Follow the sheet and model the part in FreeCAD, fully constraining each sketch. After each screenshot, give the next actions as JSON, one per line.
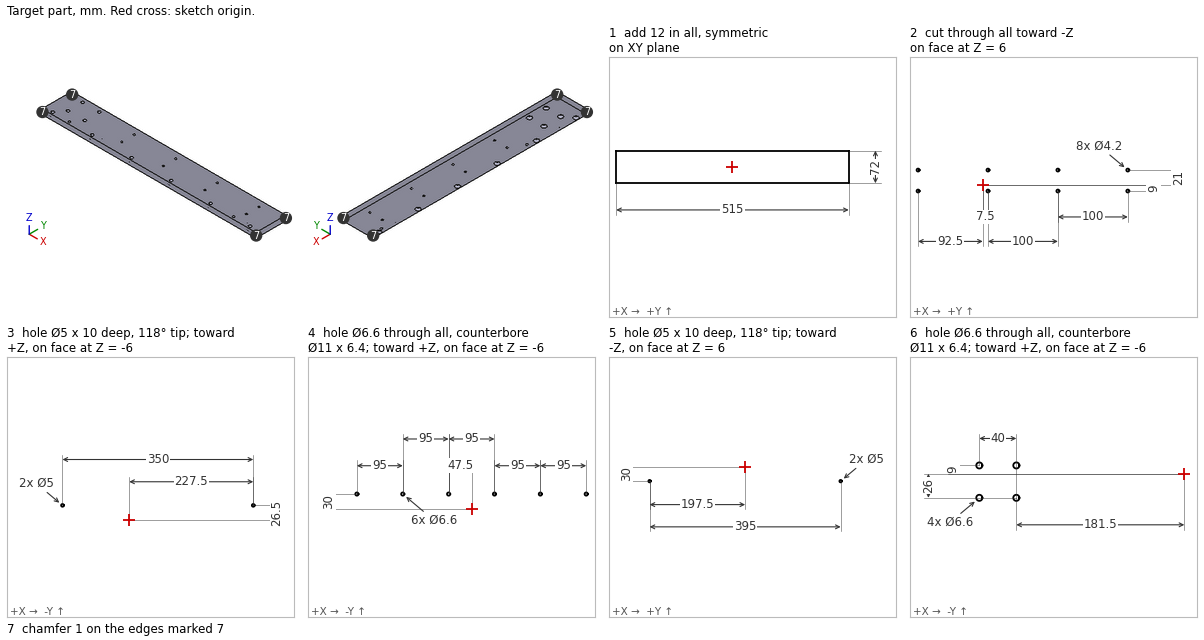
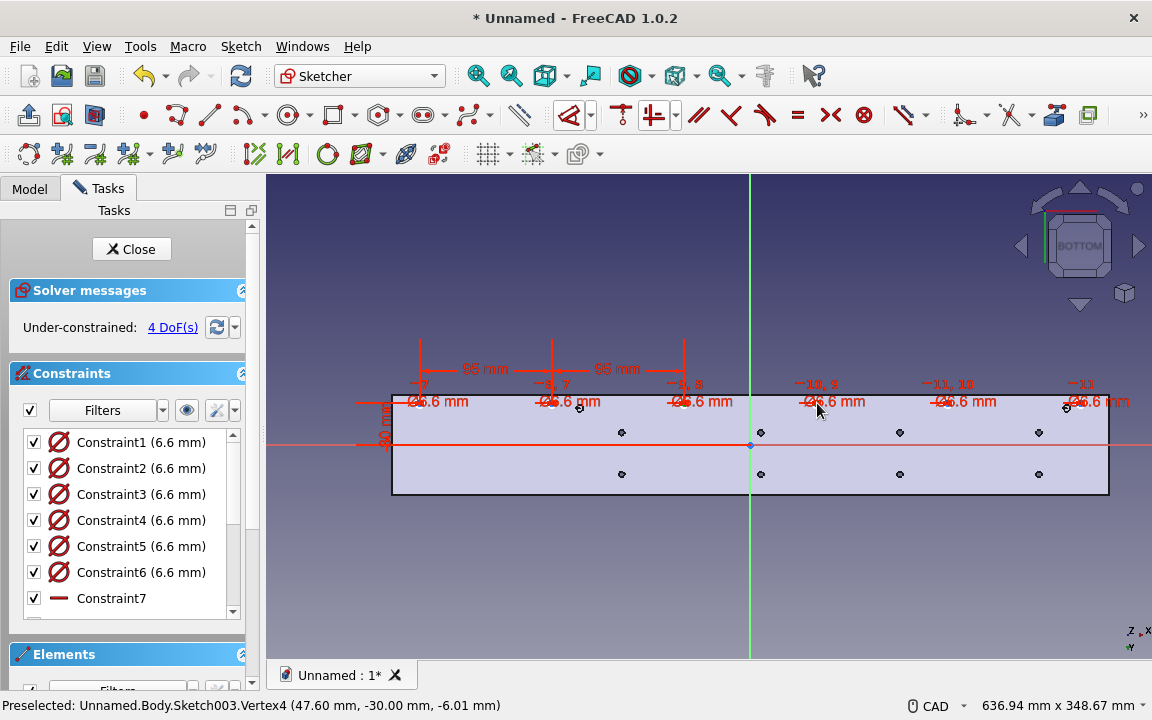
{"action": "key", "text": "l"}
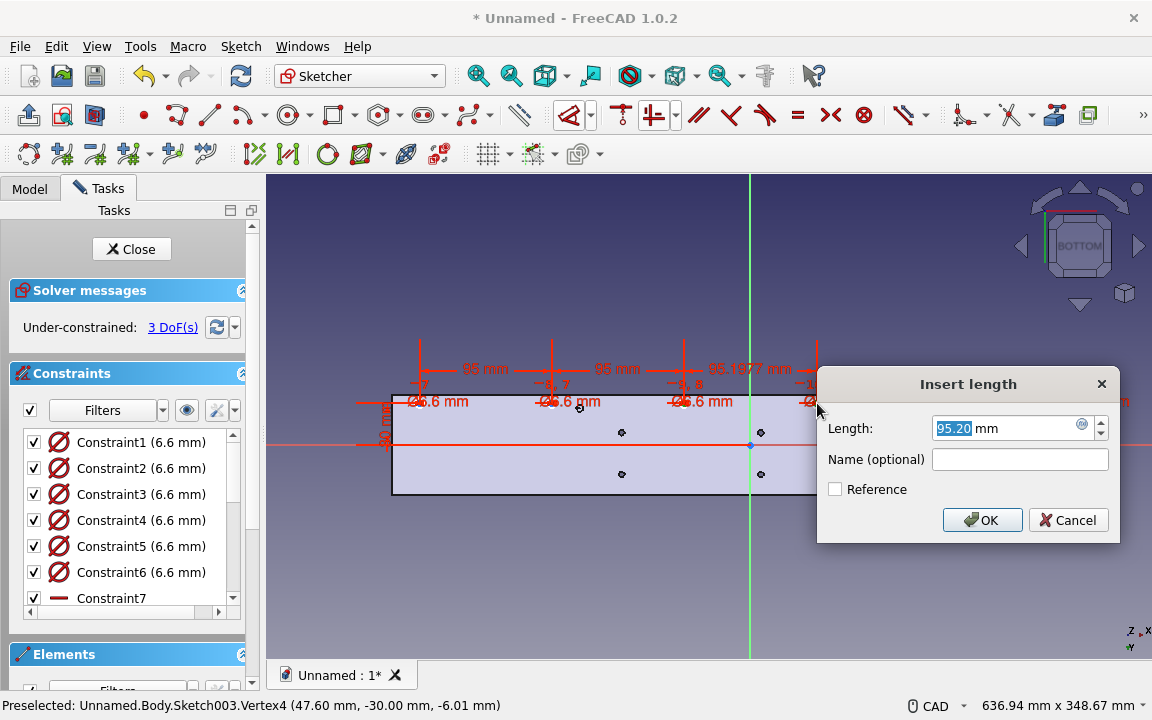
{"action": "type", "text": "95"}
{"action": "key", "text": "Return"}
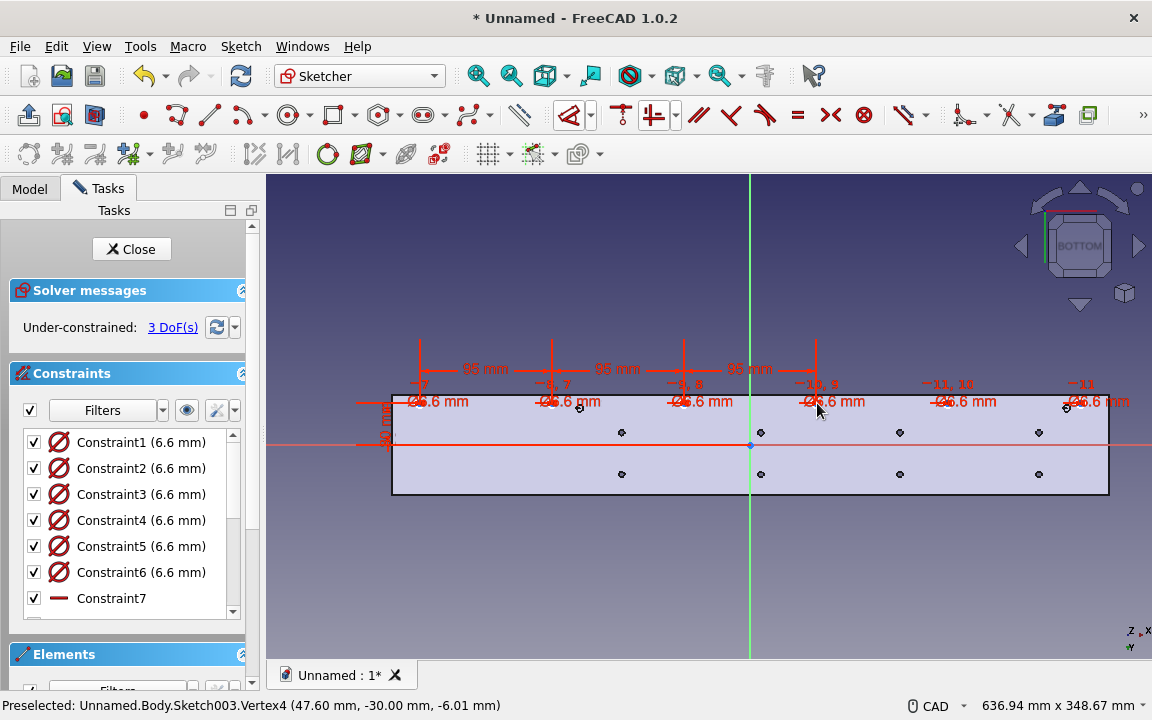
{"action": "left_click", "coordinate": [816, 403]}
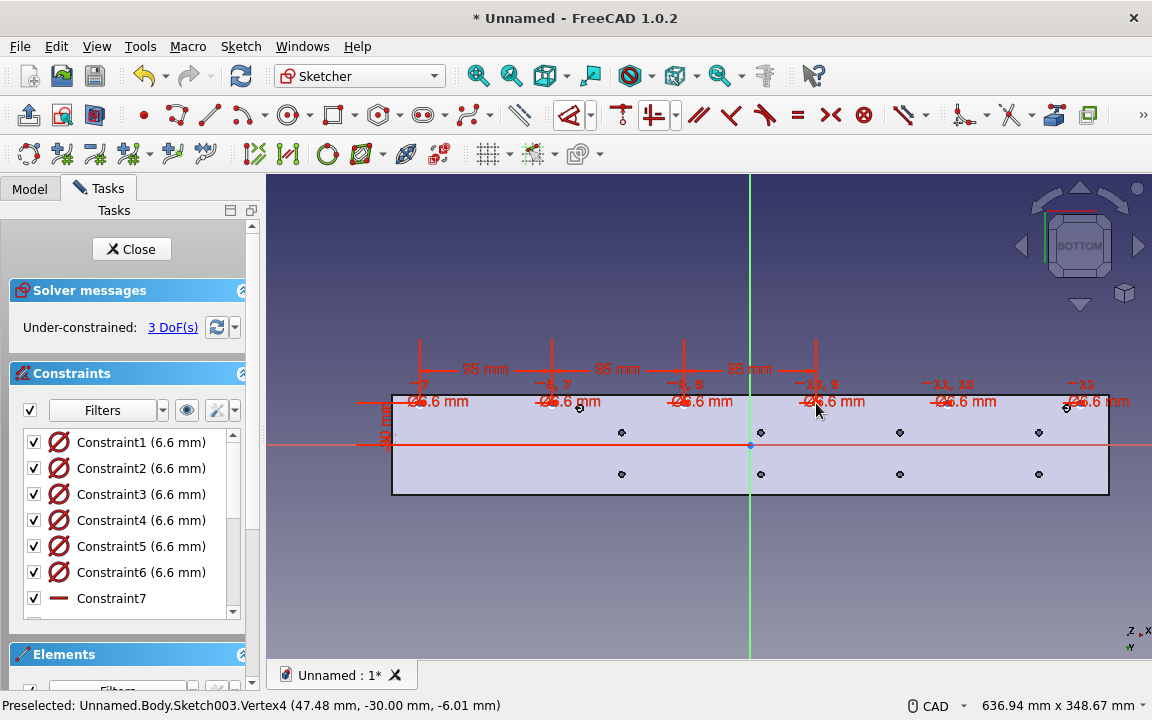
{"action": "left_click", "coordinate": [948, 403]}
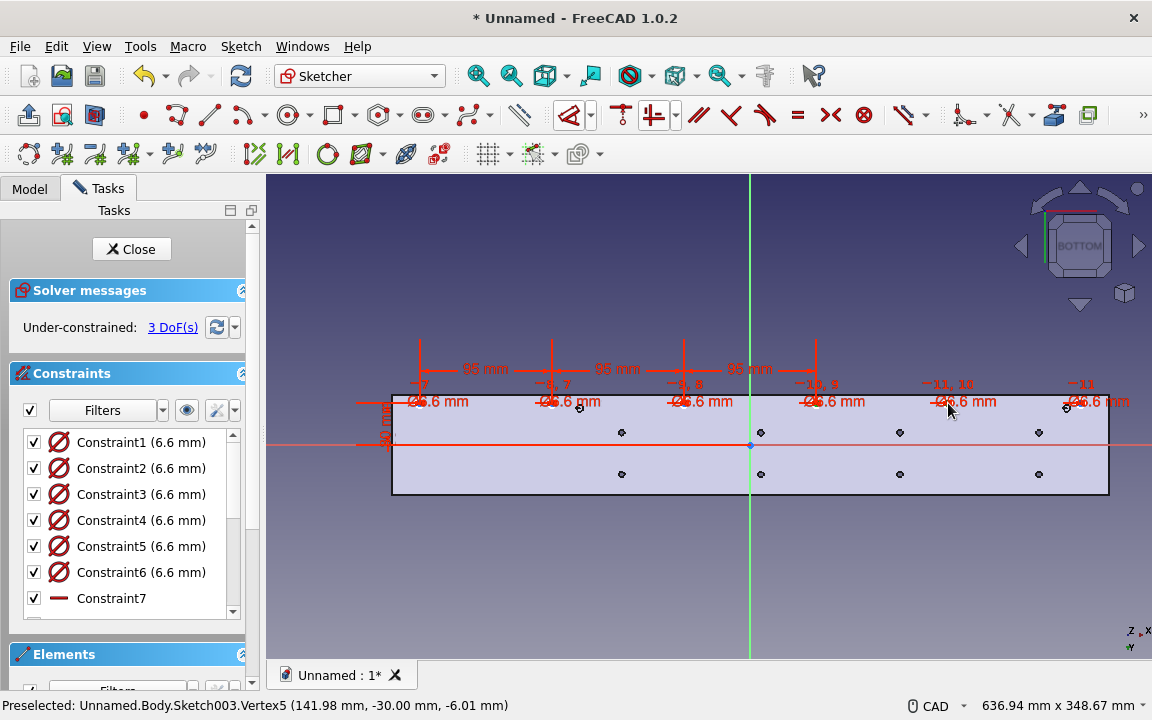
{"action": "key", "text": "l"}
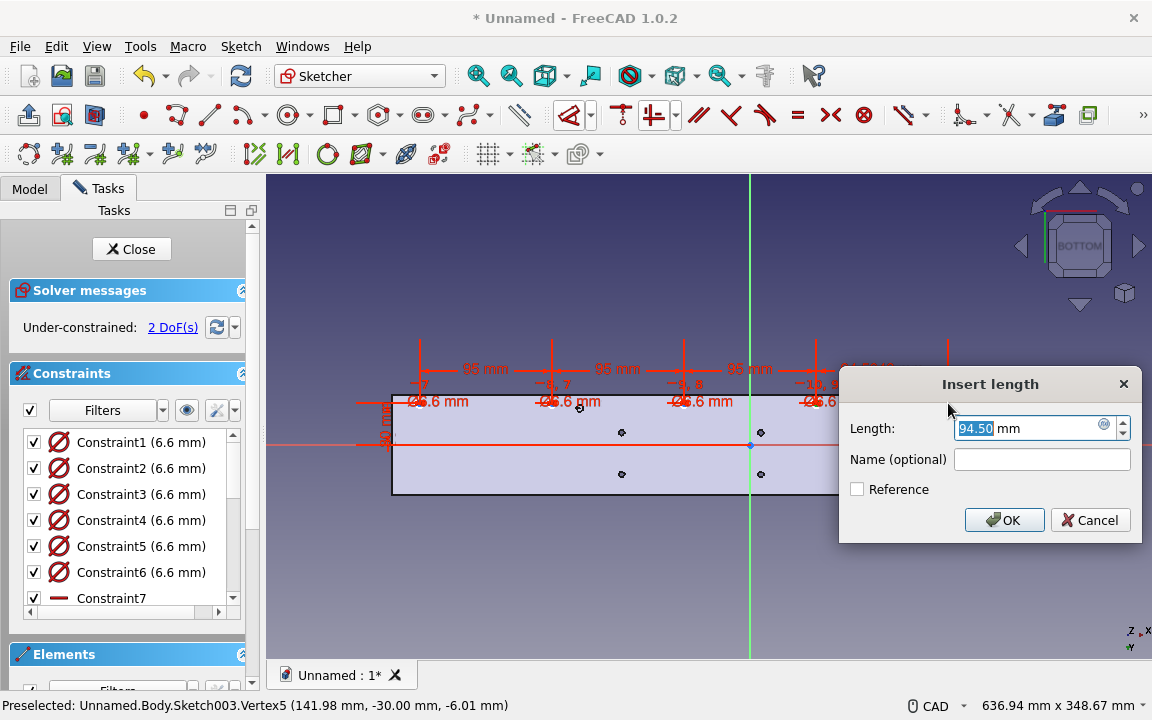
{"action": "type", "text": "95"}
{"action": "key", "text": "Return"}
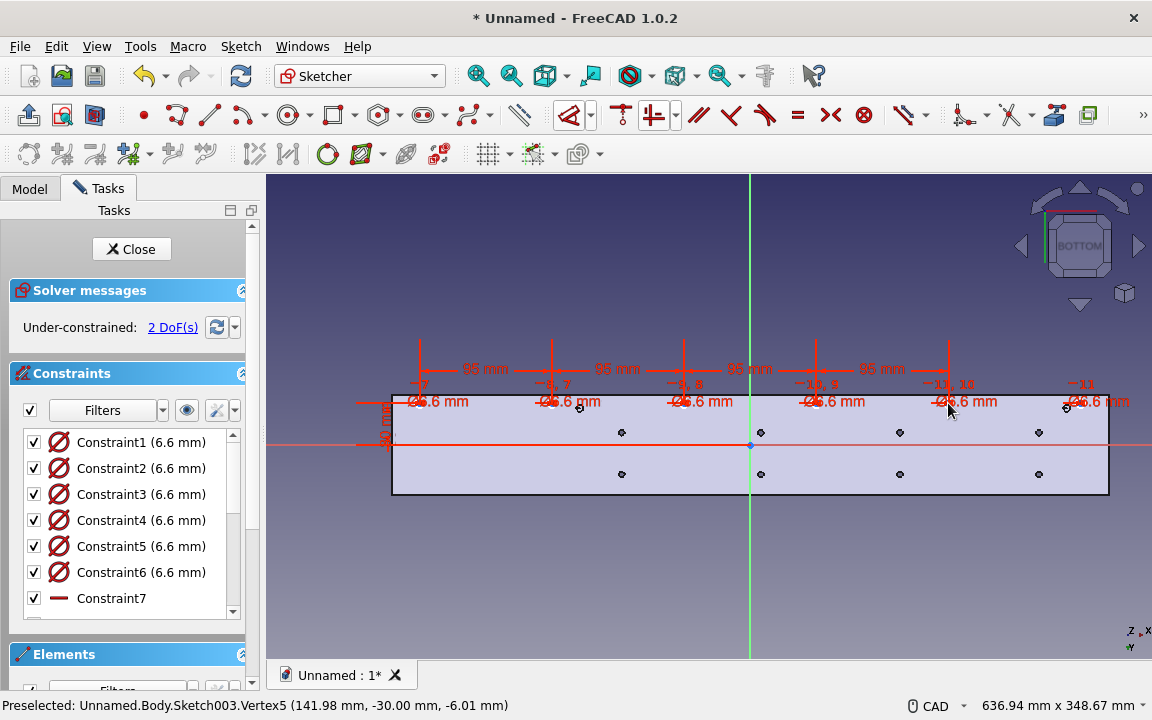
{"action": "left_click", "coordinate": [949, 403]}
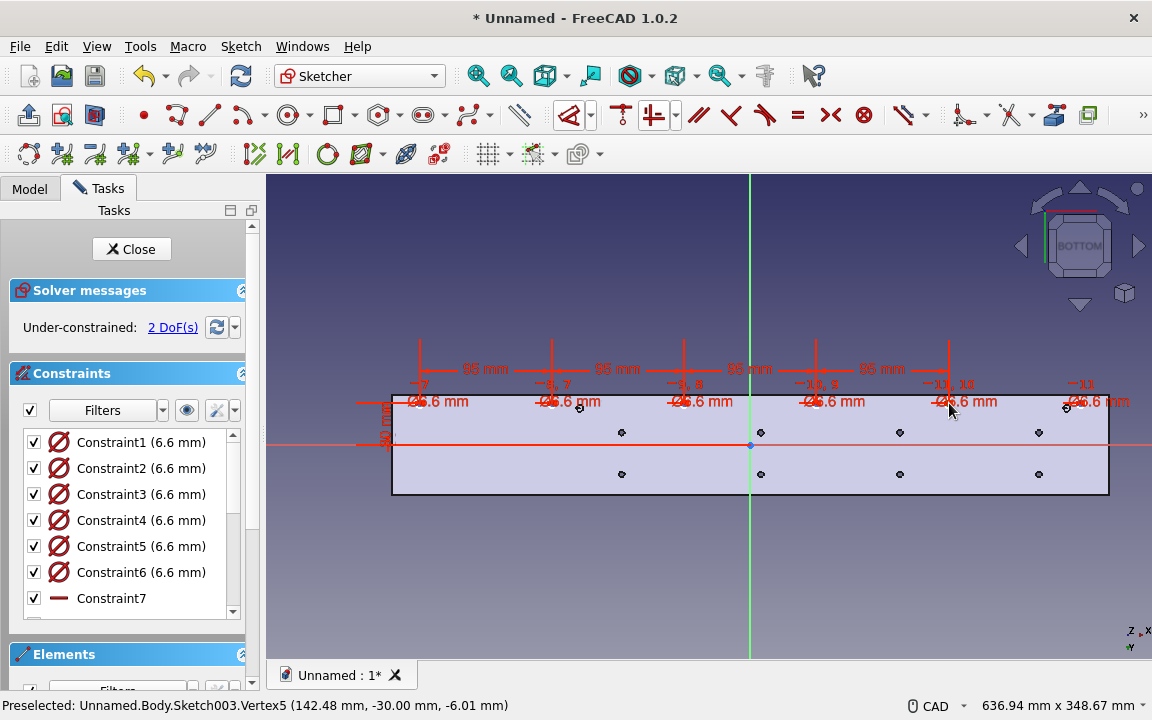
{"action": "scroll", "coordinate": [417, 405], "scroll_direction": "down", "scroll_amount": 2}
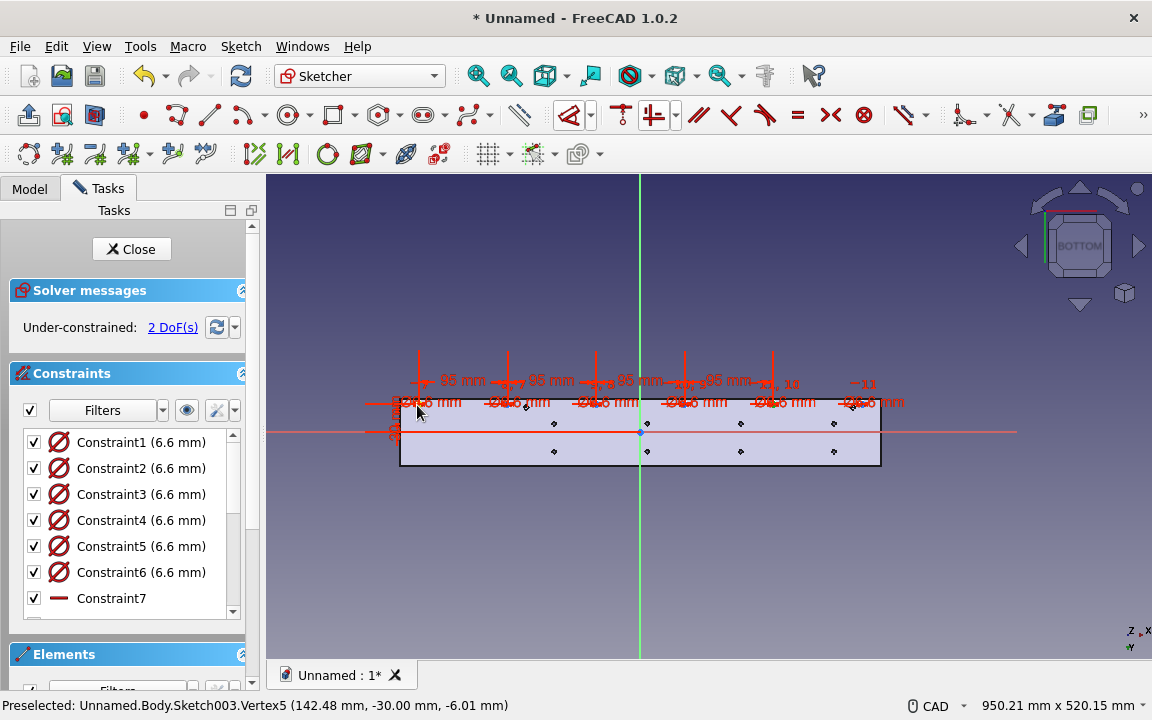
{"action": "left_click", "coordinate": [862, 404]}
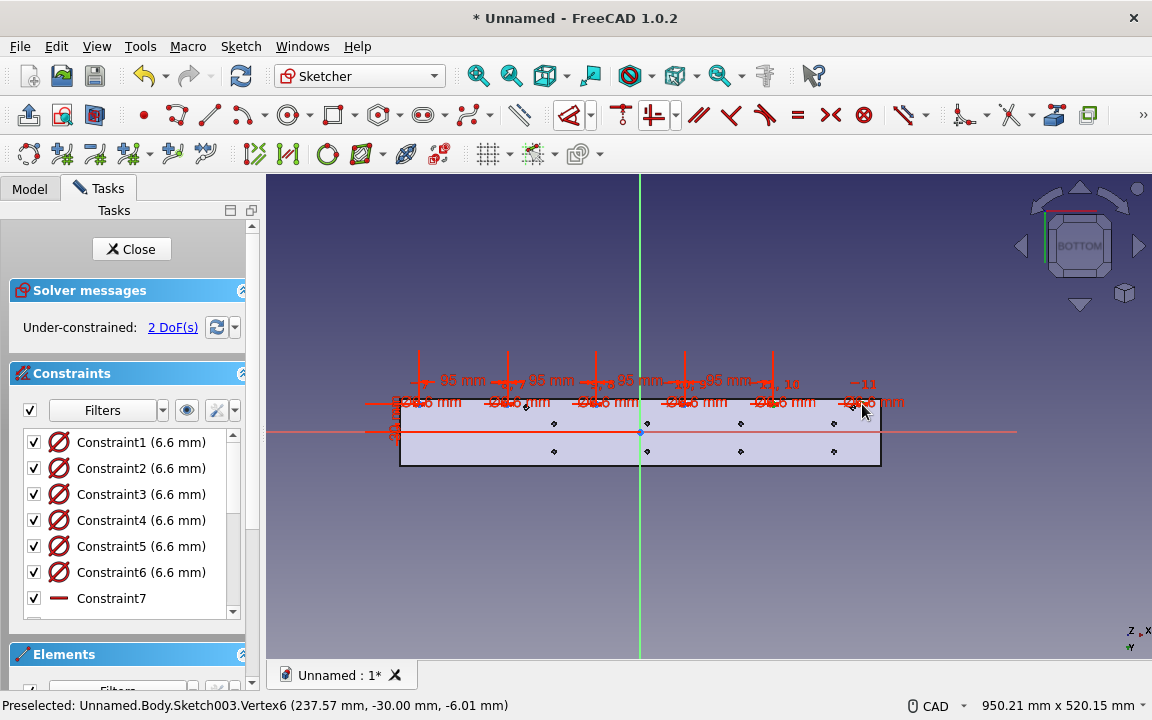
{"action": "left_click", "coordinate": [590, 116]}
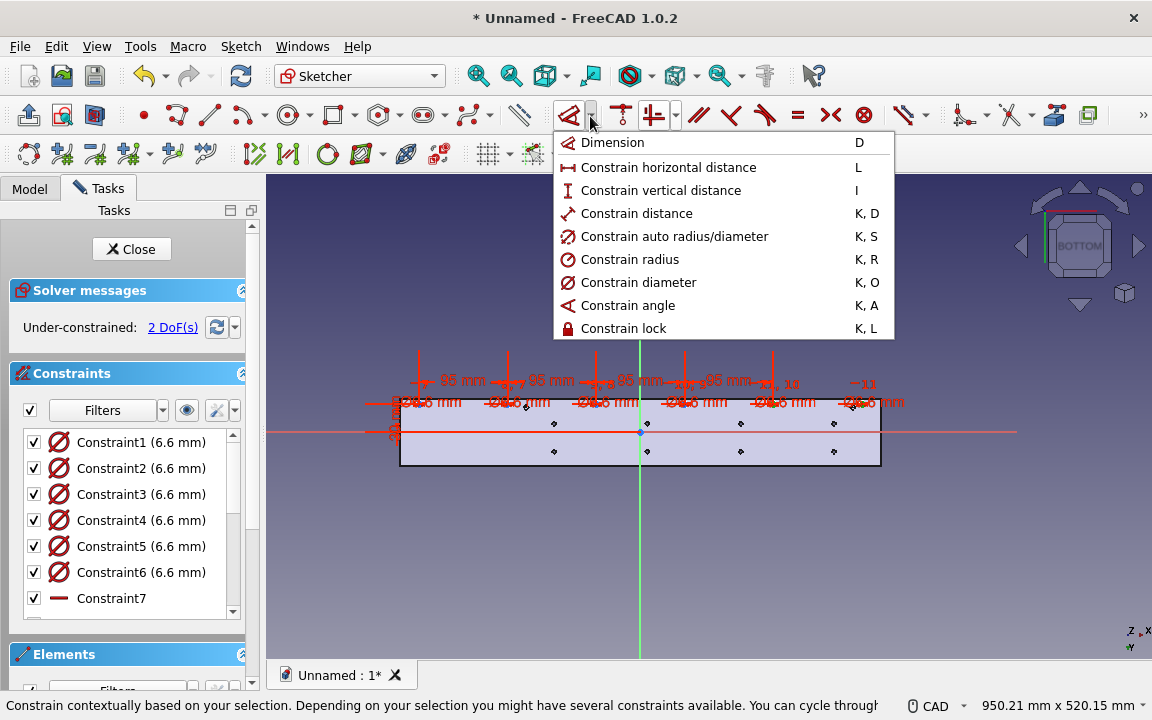
{"action": "left_click", "coordinate": [724, 168]}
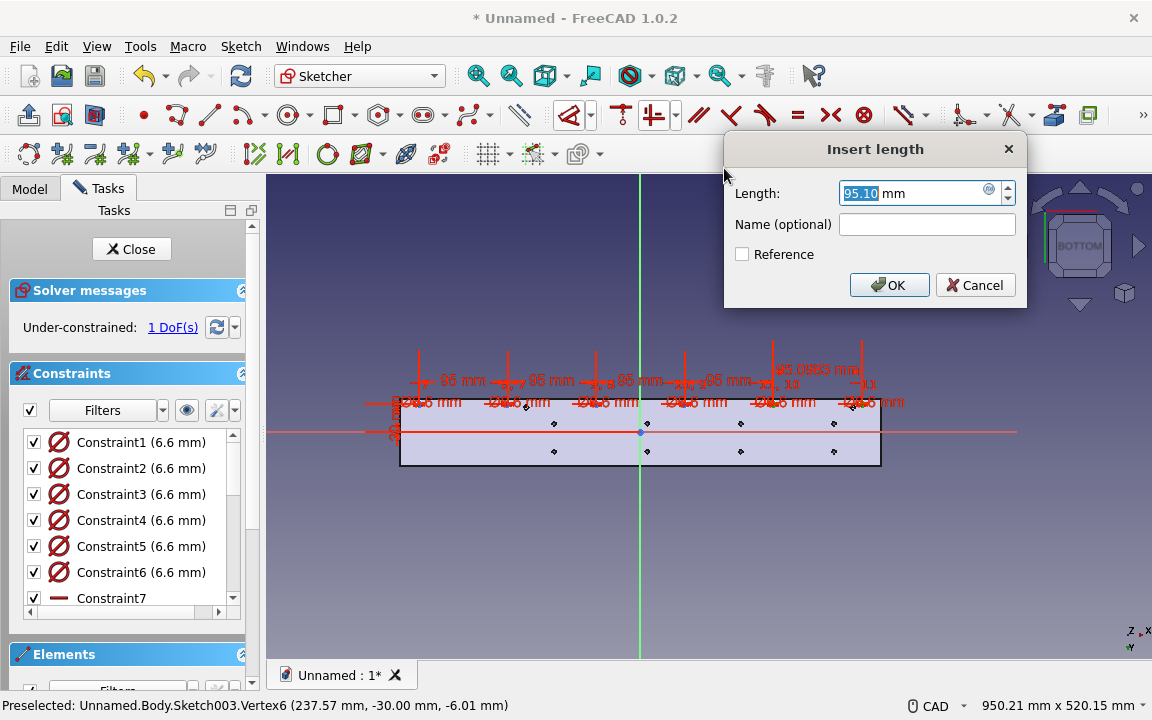
{"action": "type", "text": "95"}
{"action": "key", "text": "Return"}